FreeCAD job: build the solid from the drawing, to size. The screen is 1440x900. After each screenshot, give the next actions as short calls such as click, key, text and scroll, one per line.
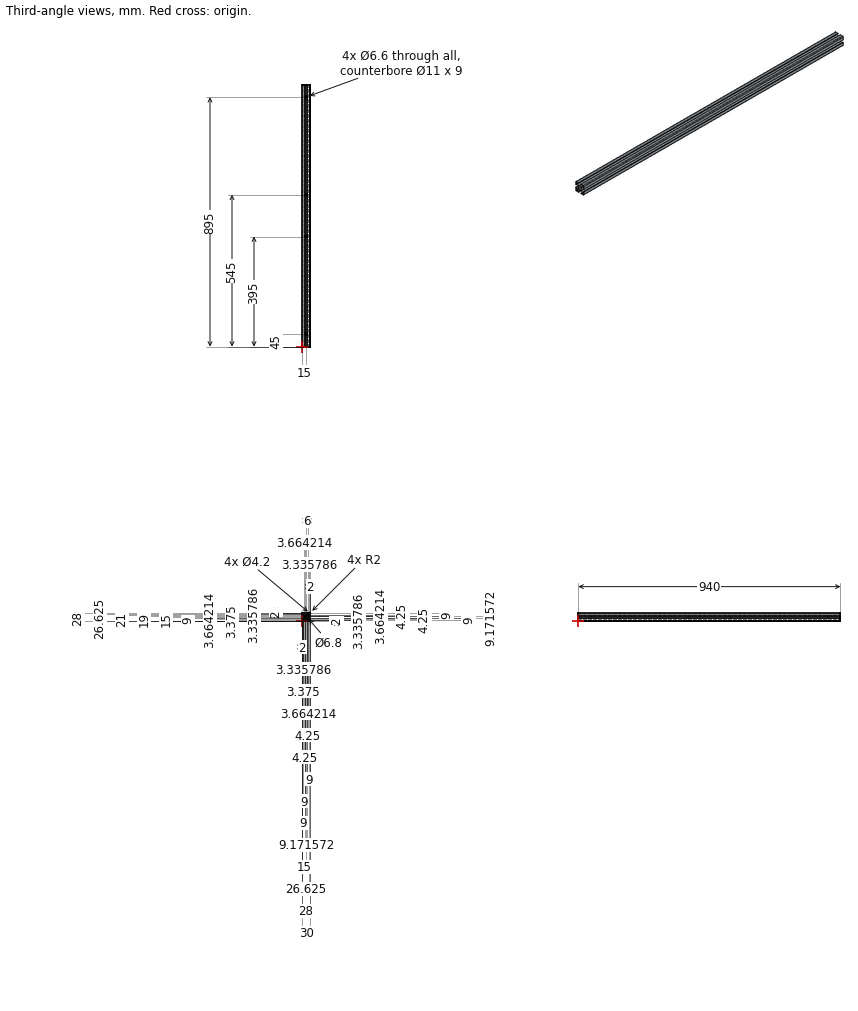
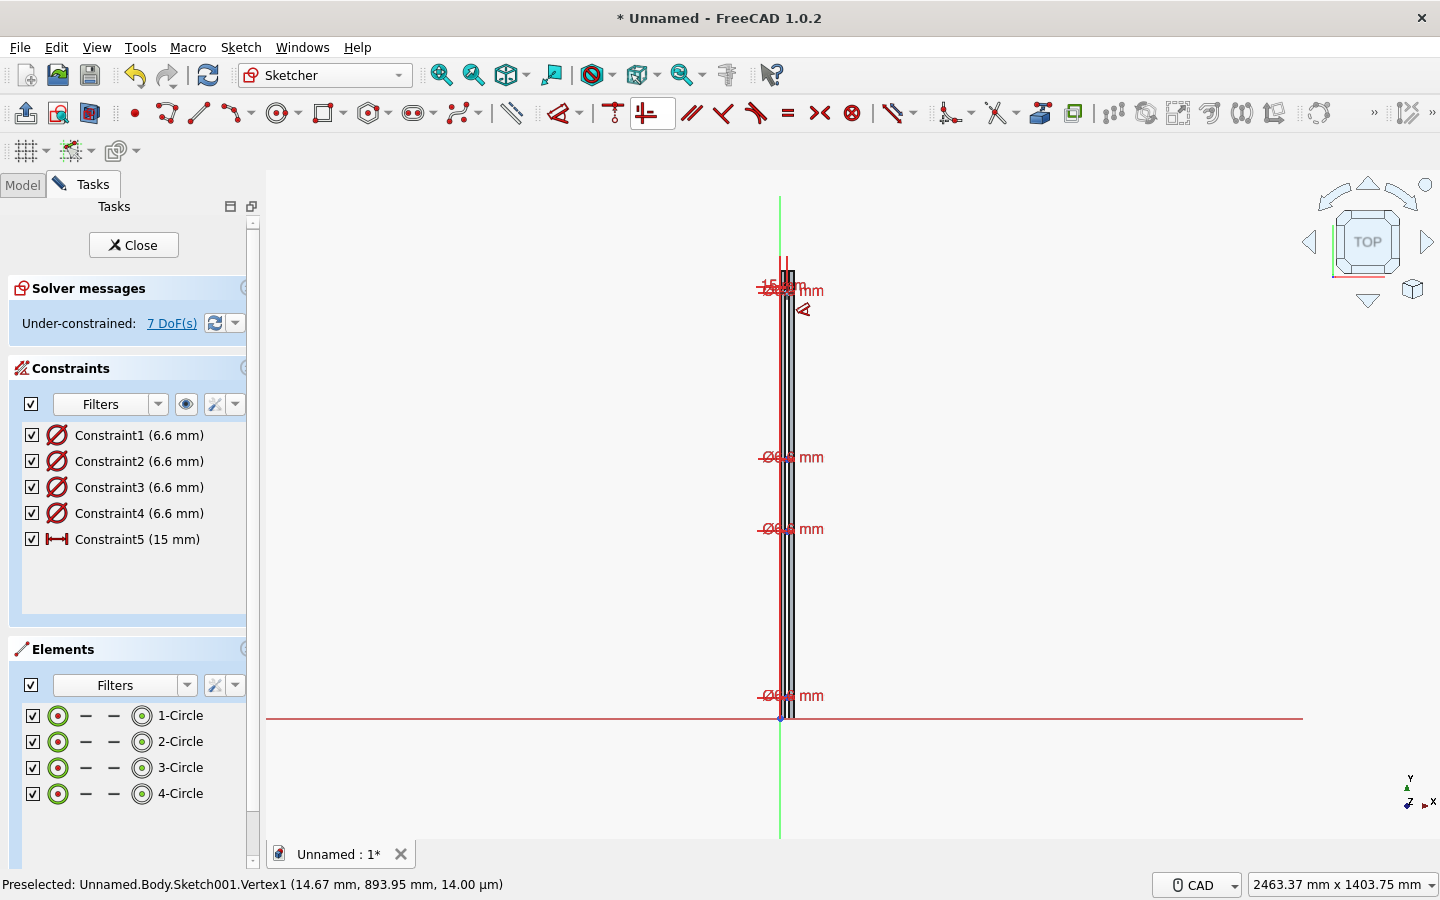
scroll(787, 459, up, 9)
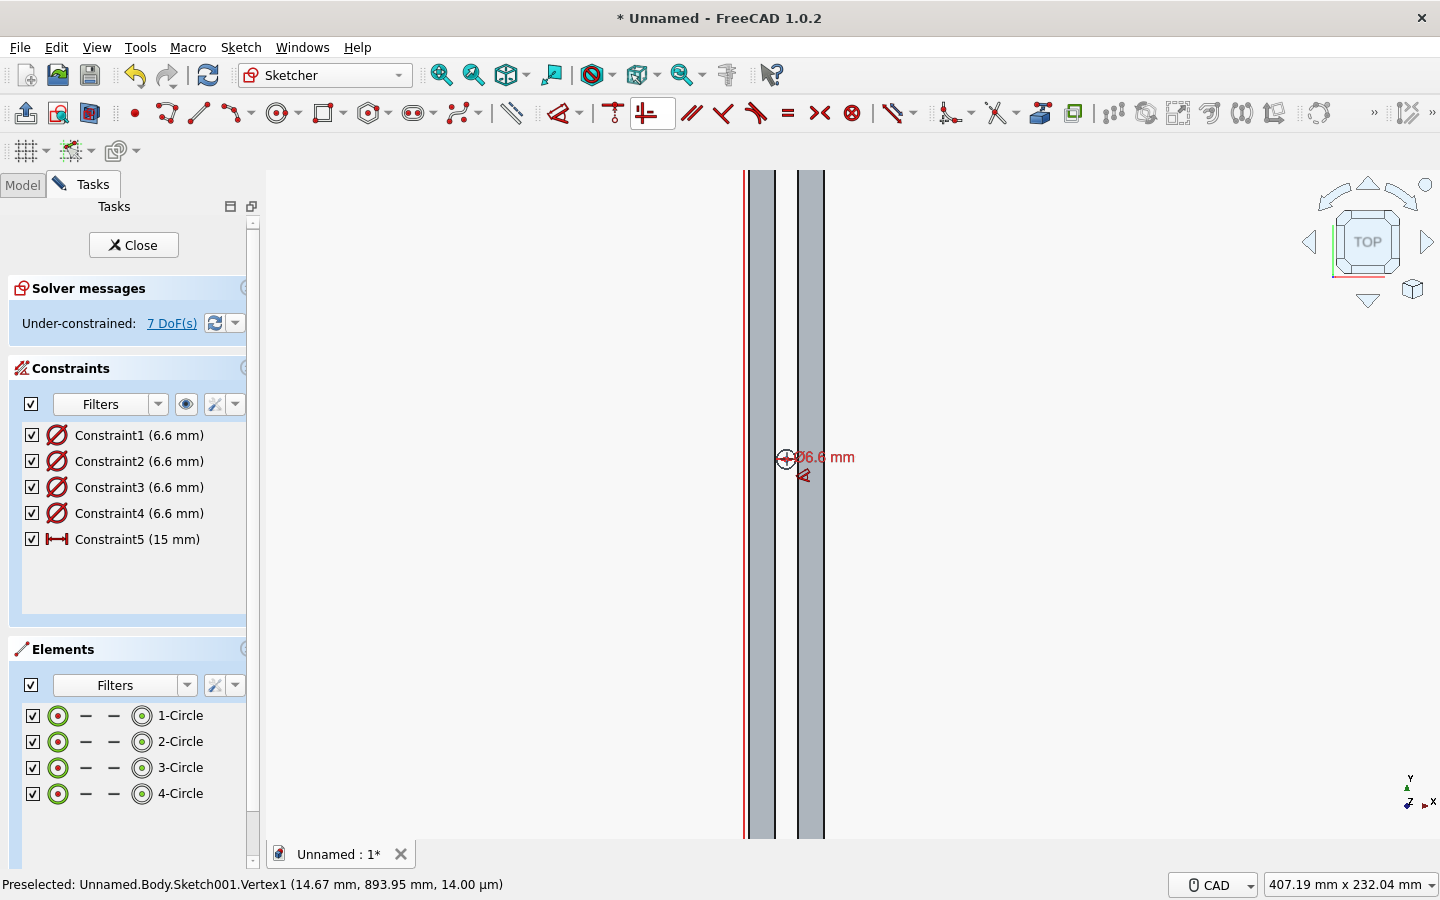
click(786, 459)
click(765, 425)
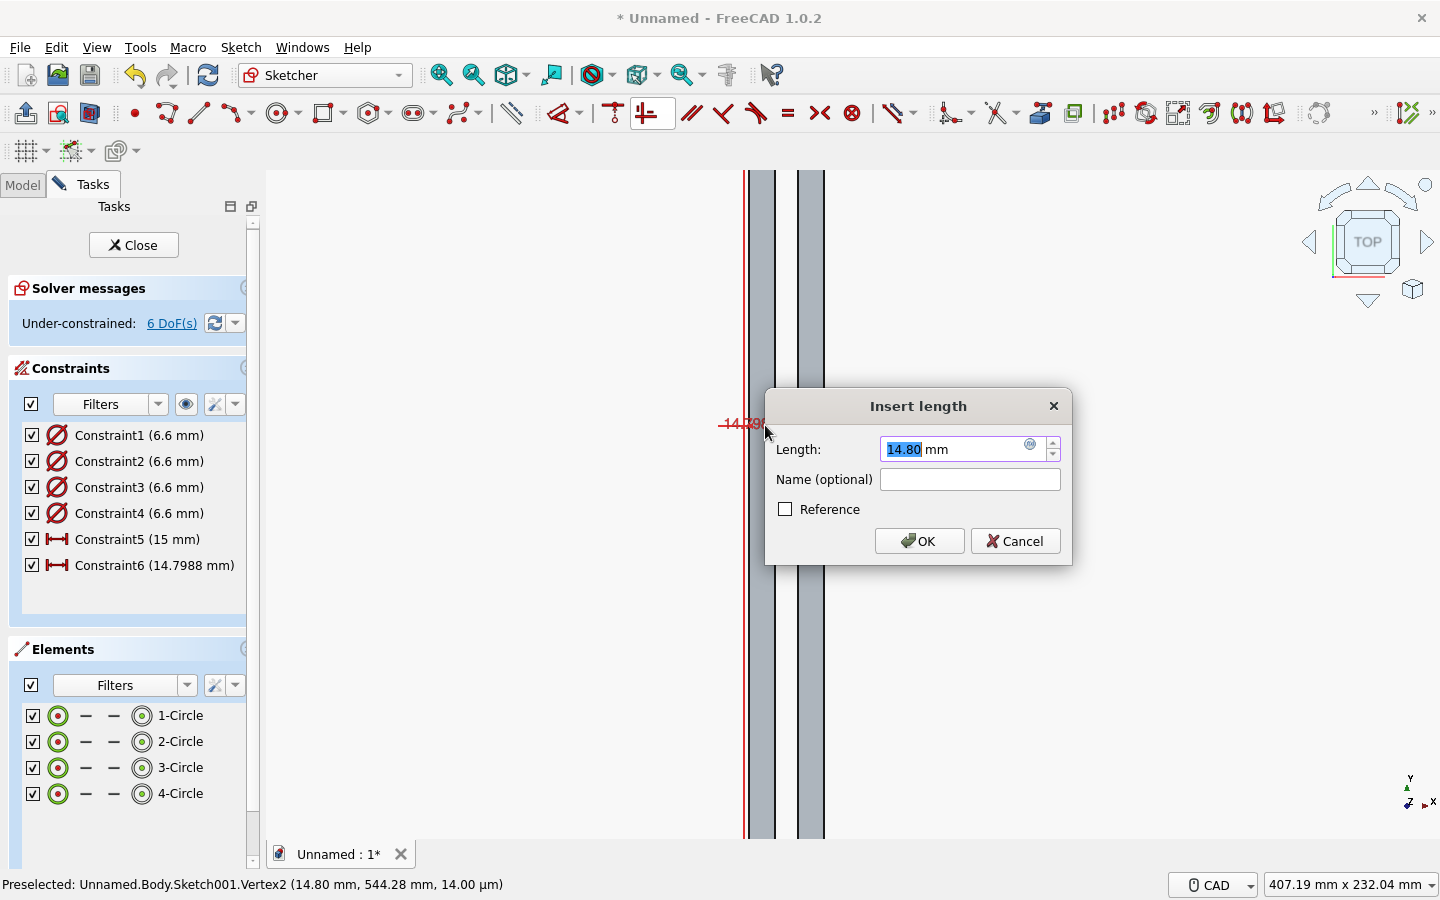
text(15)
key(Return)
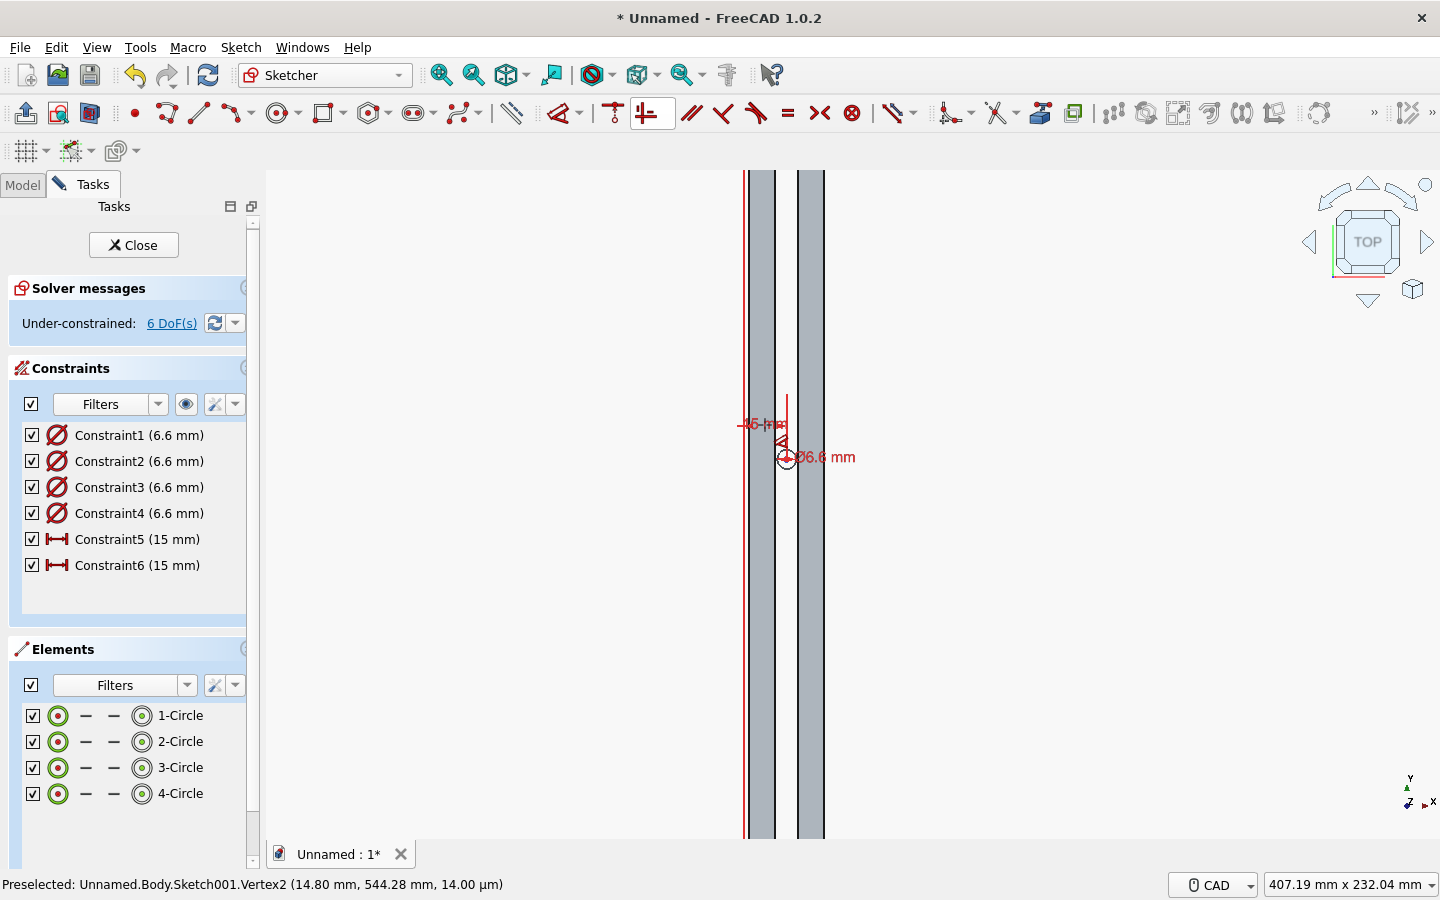
scroll(787, 459, down, 9)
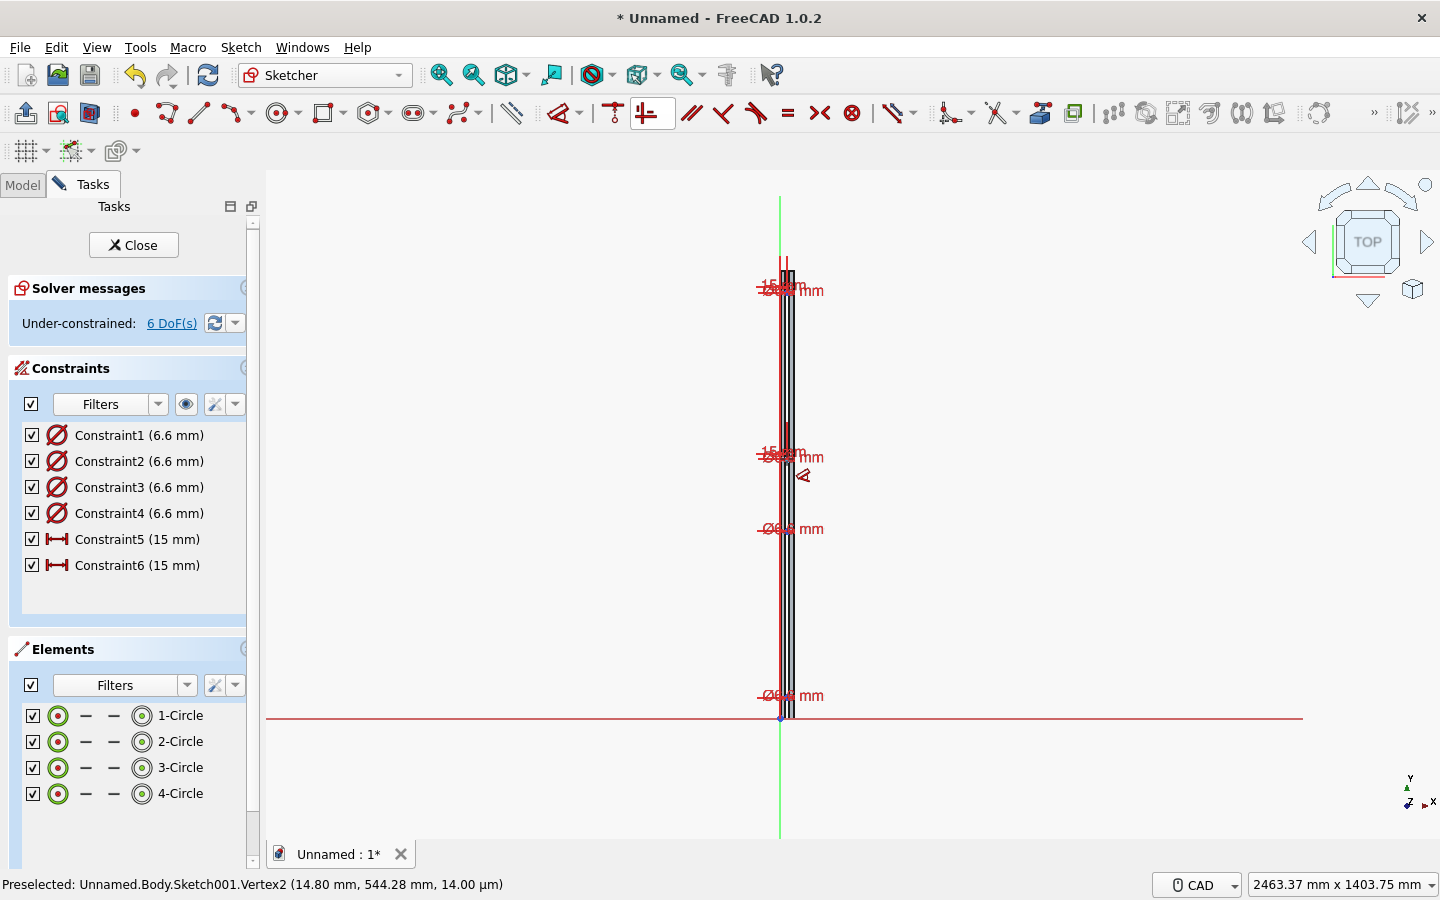
scroll(787, 698, up, 9)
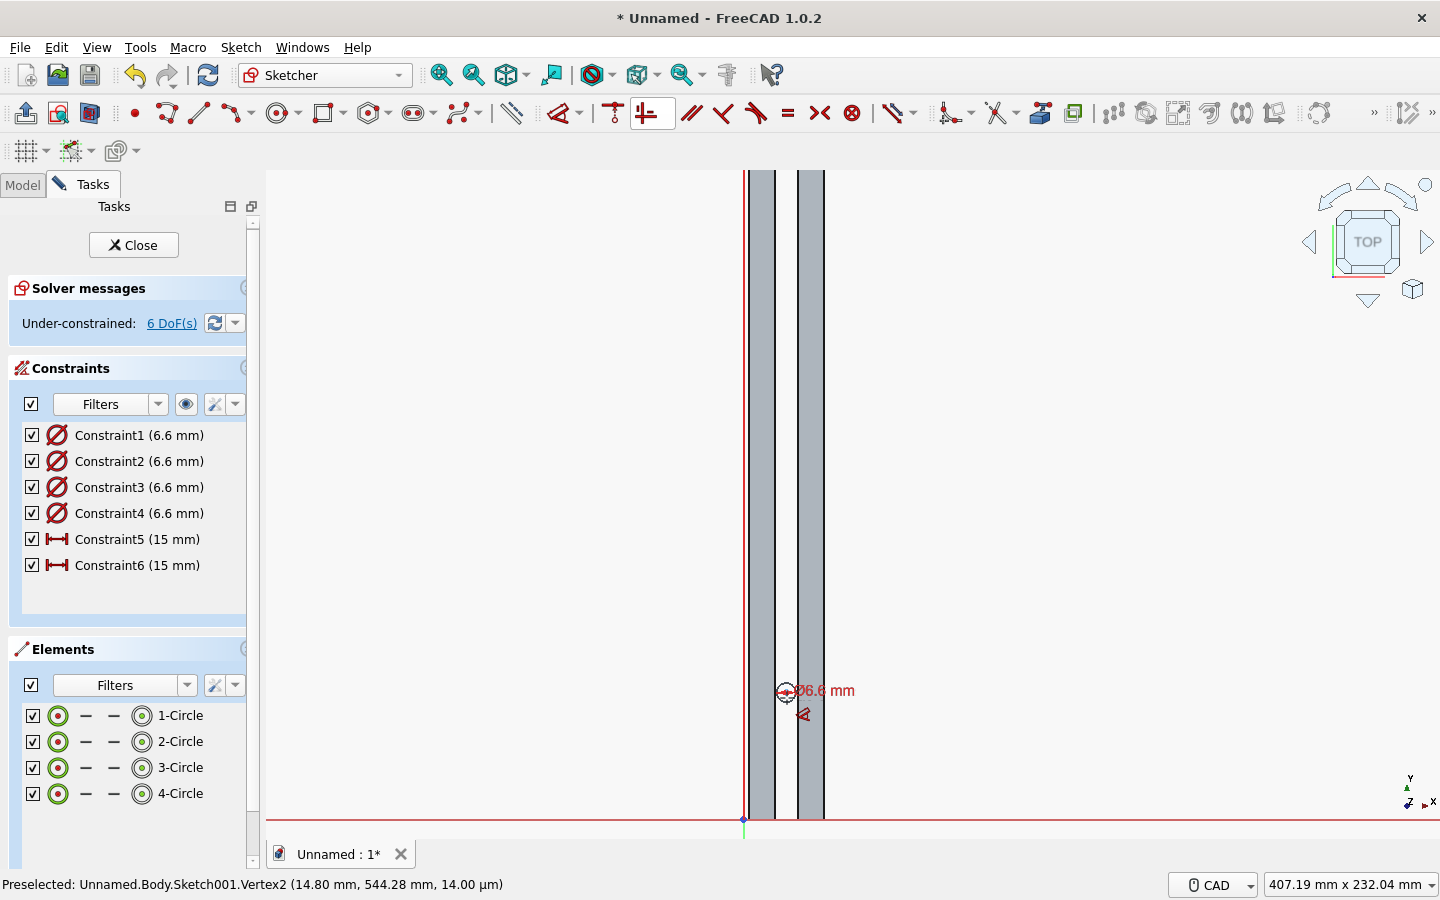
click(786, 693)
click(765, 659)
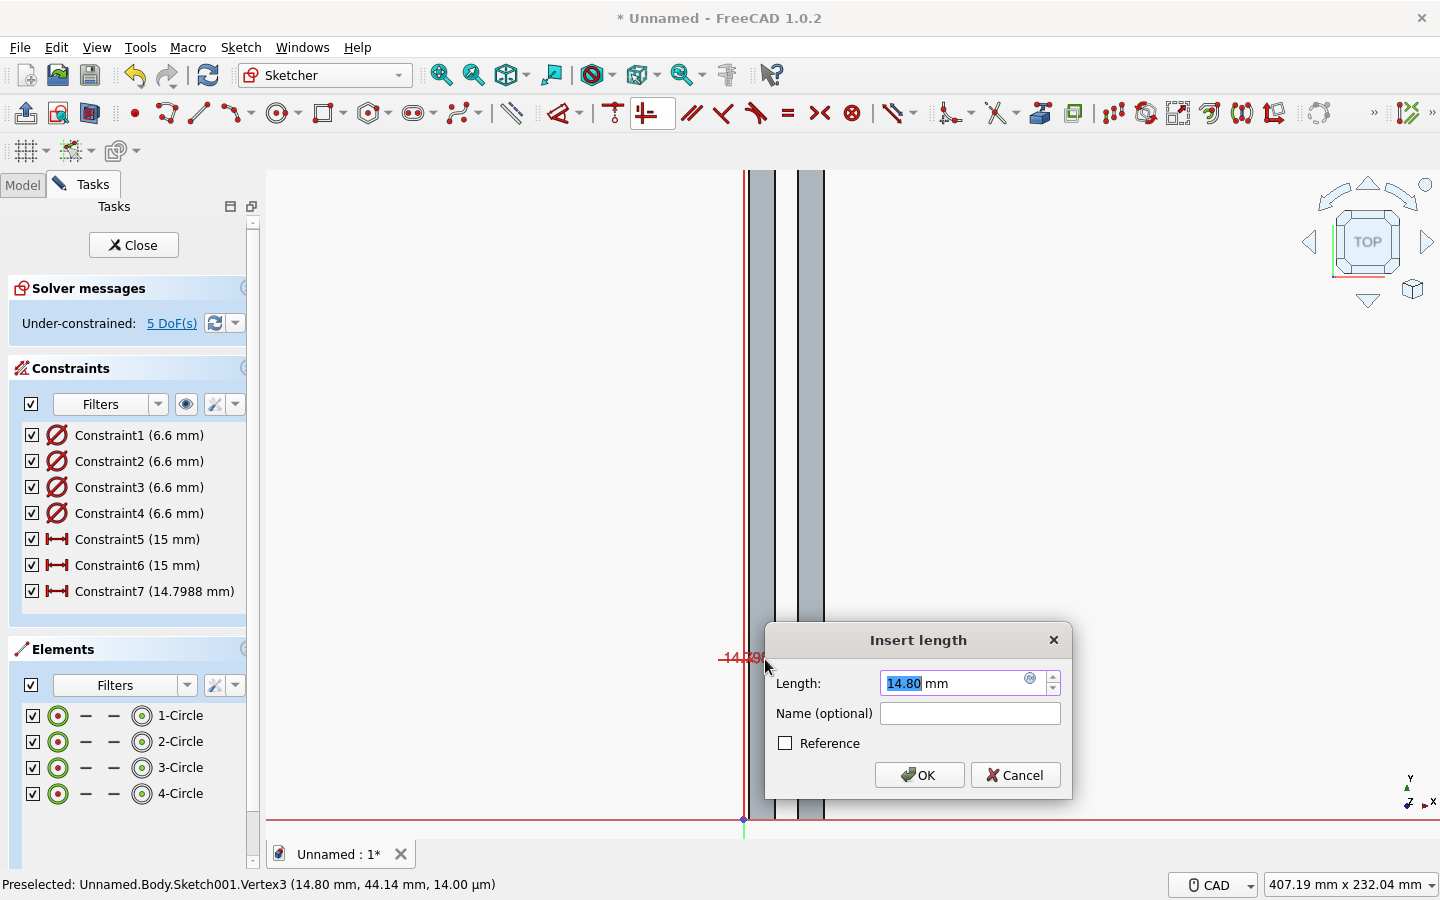
text(15)
key(Return)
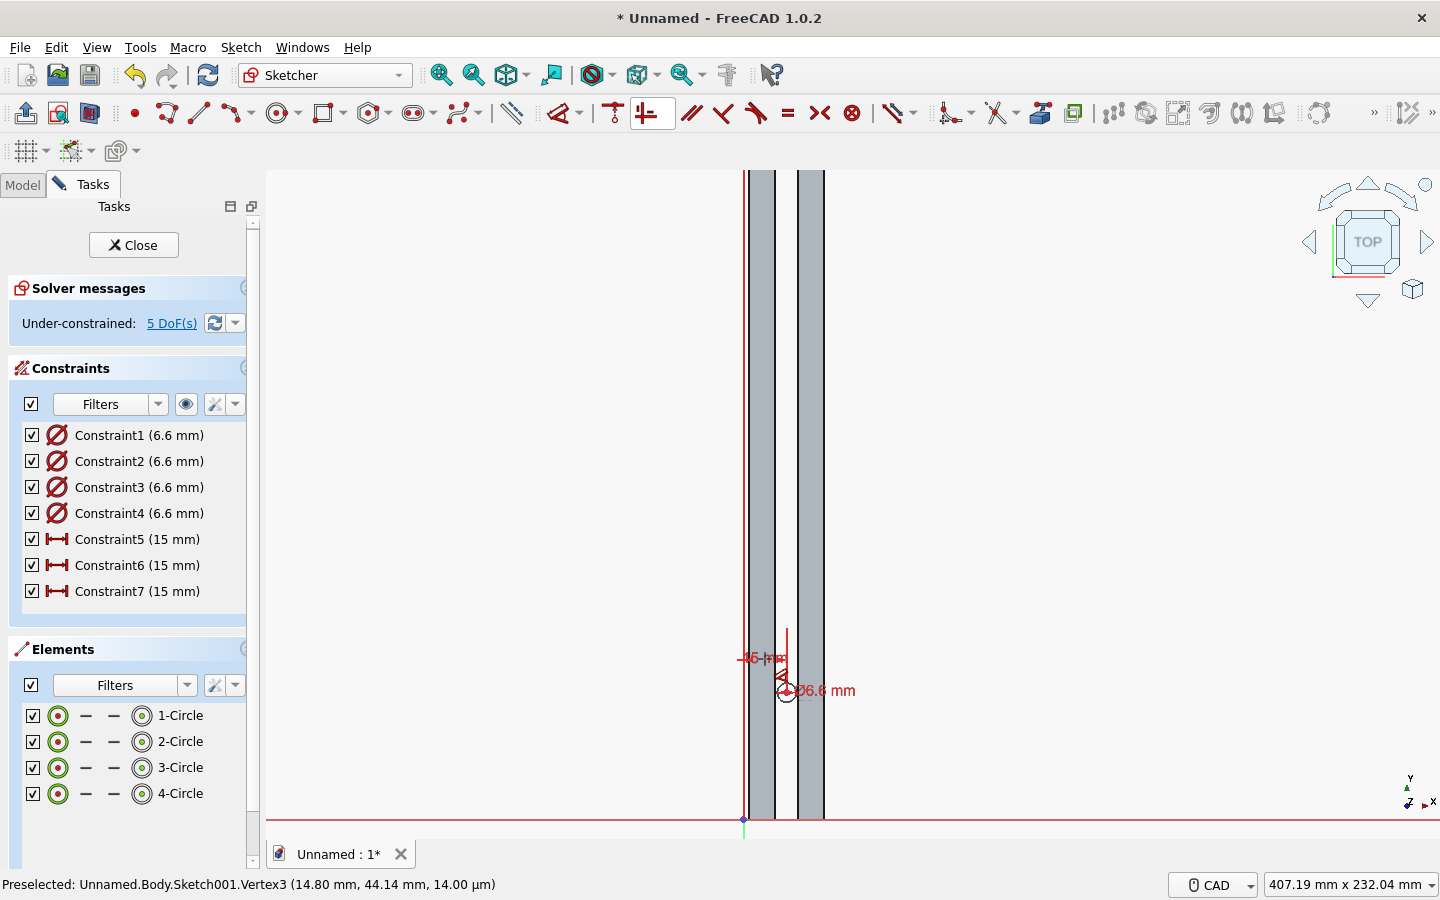
scroll(787, 698, down, 9)